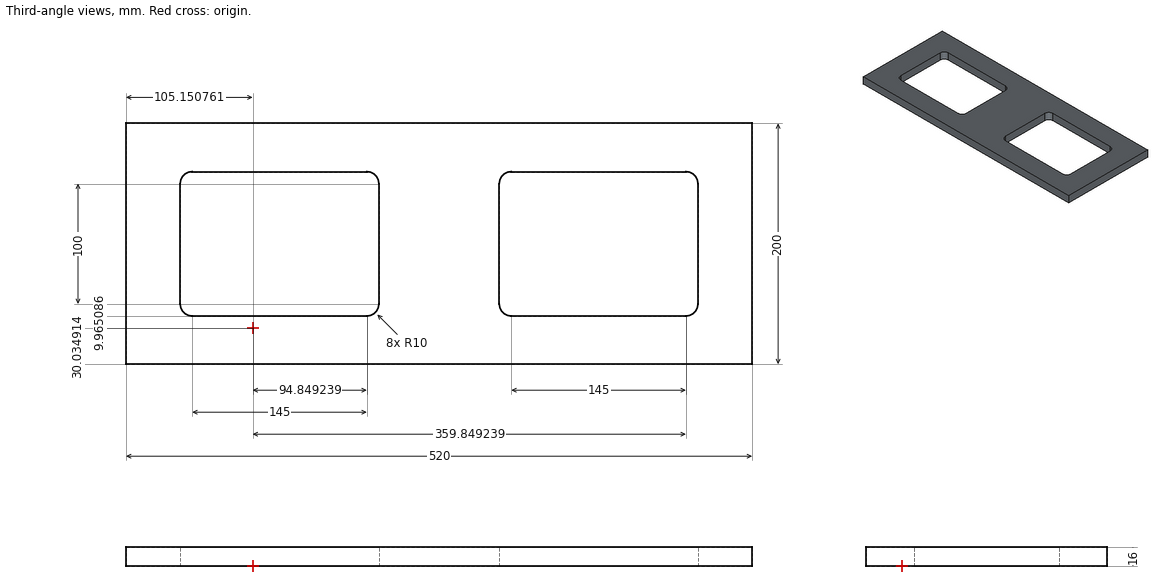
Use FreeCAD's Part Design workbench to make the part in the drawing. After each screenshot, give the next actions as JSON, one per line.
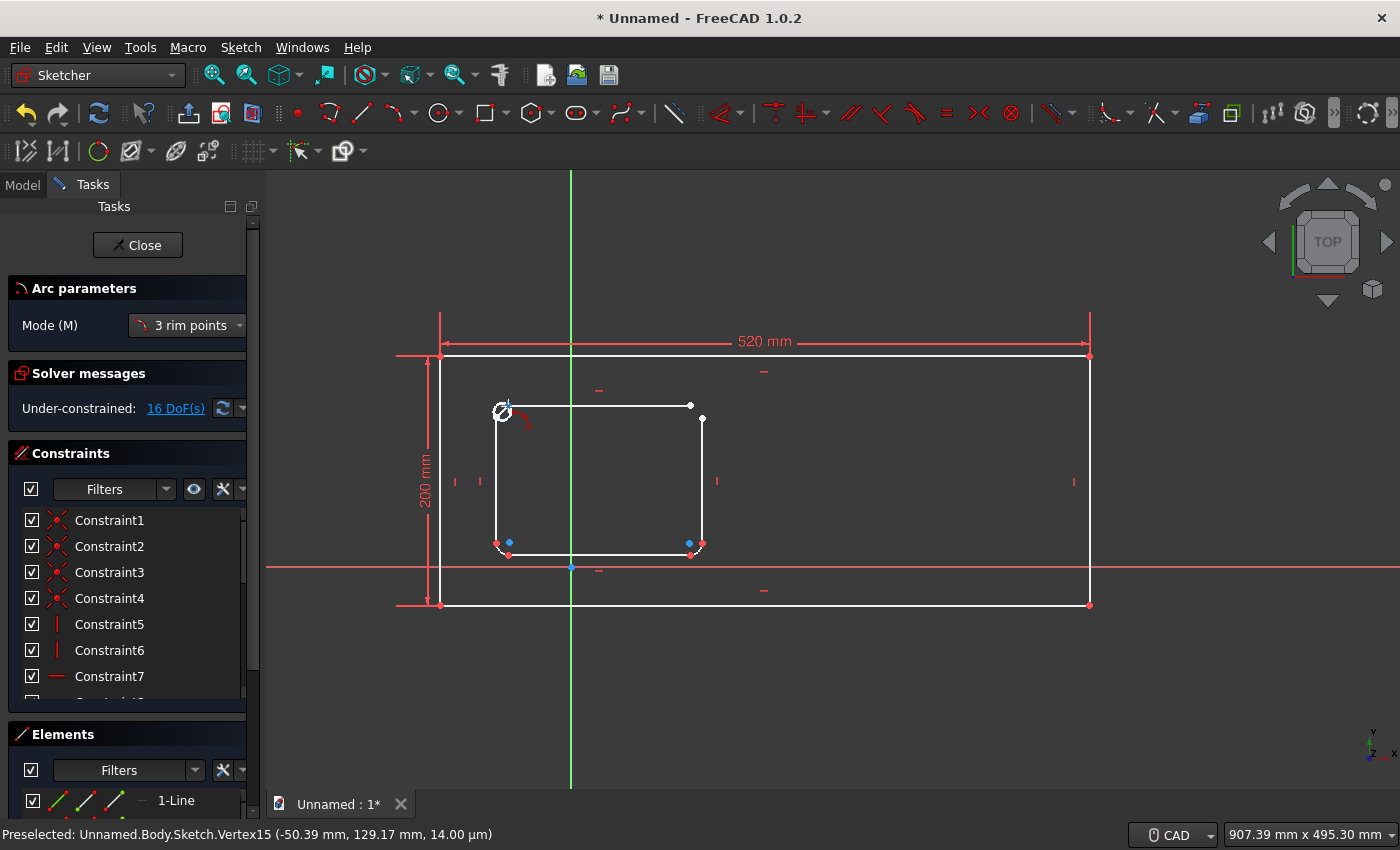
{"action": "scroll", "coordinate": [500, 408], "scroll_direction": "up", "scroll_amount": 8}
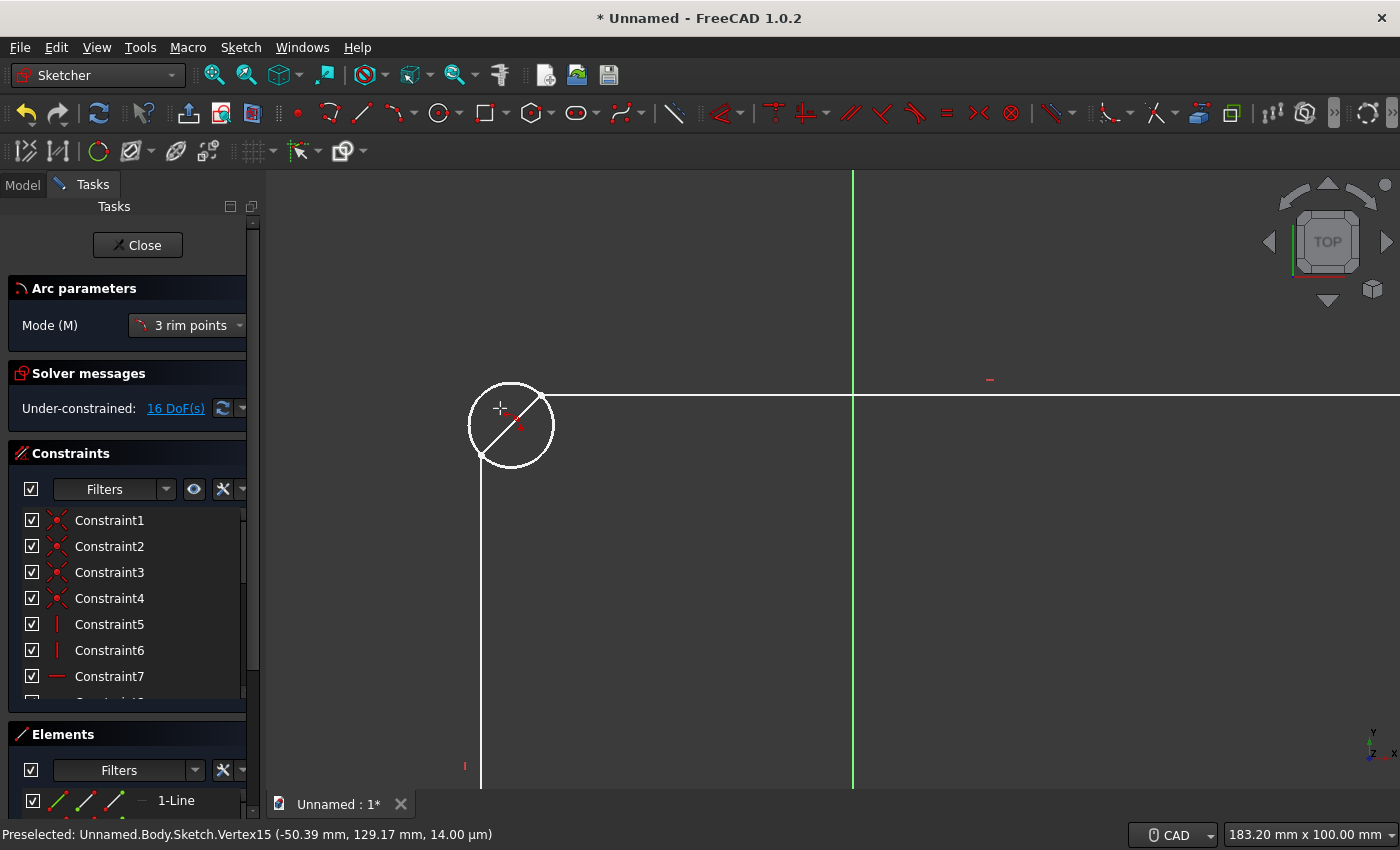
{"action": "left_click", "coordinate": [499, 409]}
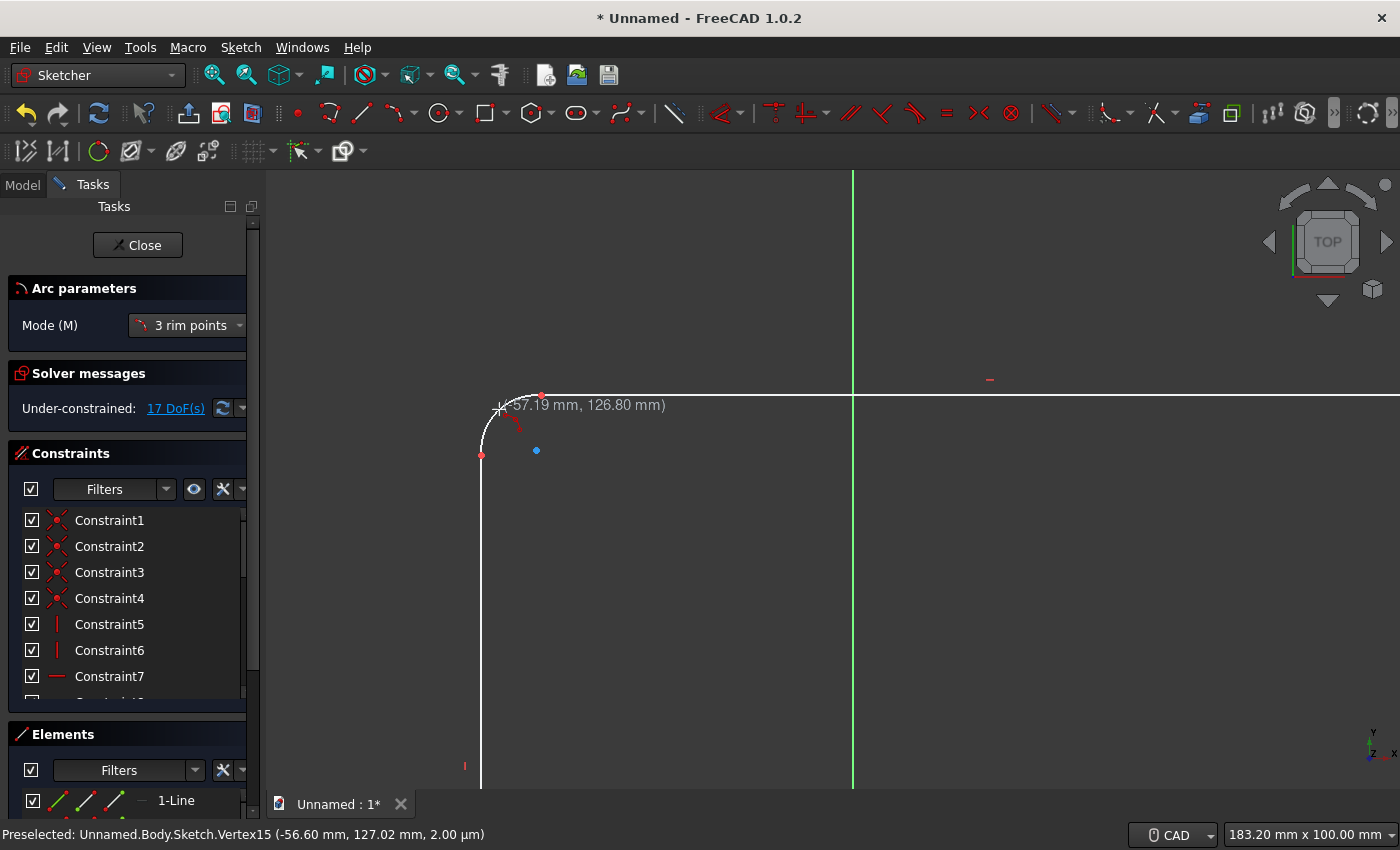
{"action": "scroll", "coordinate": [500, 408], "scroll_direction": "down", "scroll_amount": 8}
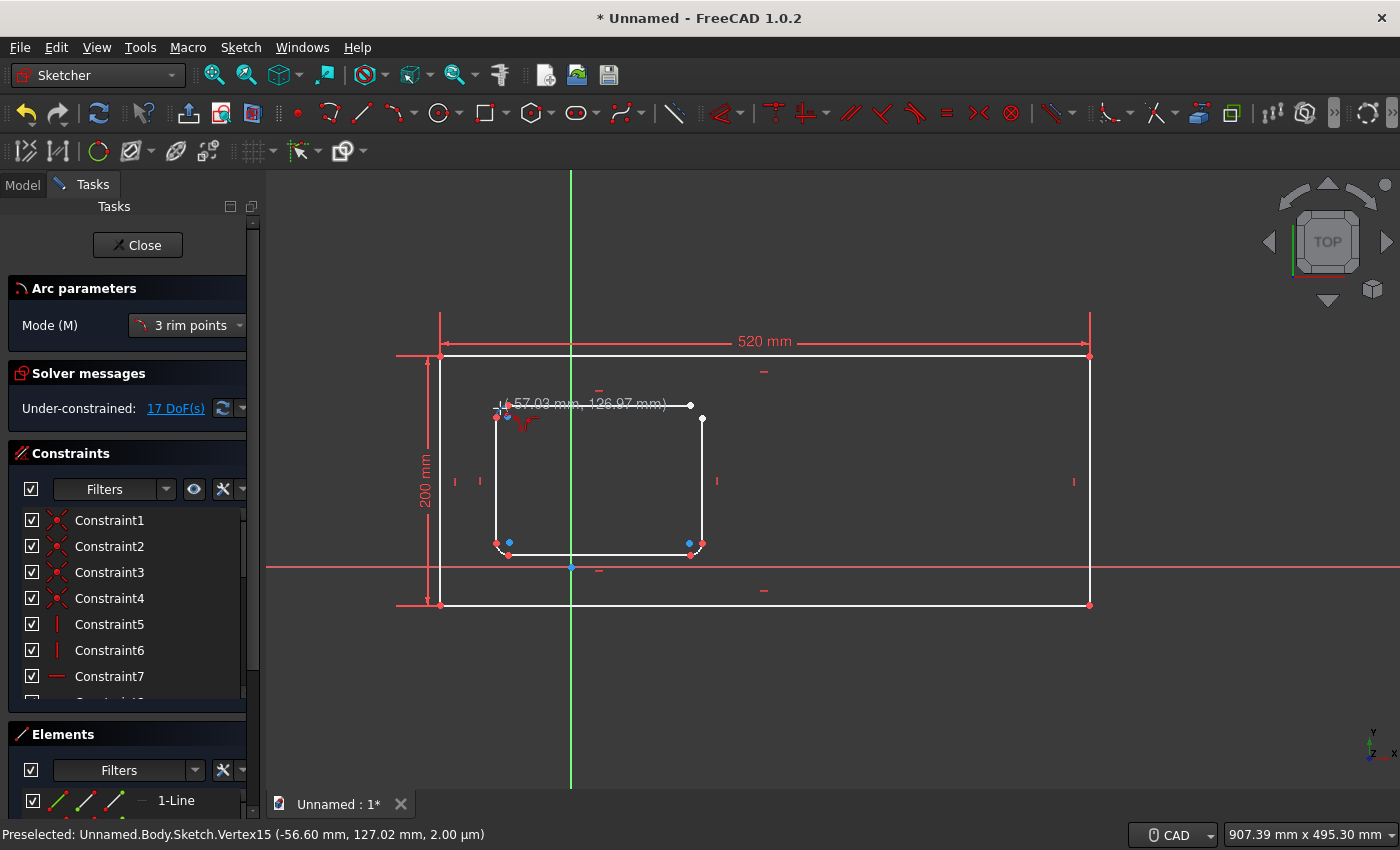
{"action": "left_click", "coordinate": [690, 406]}
{"action": "left_click", "coordinate": [702, 418]}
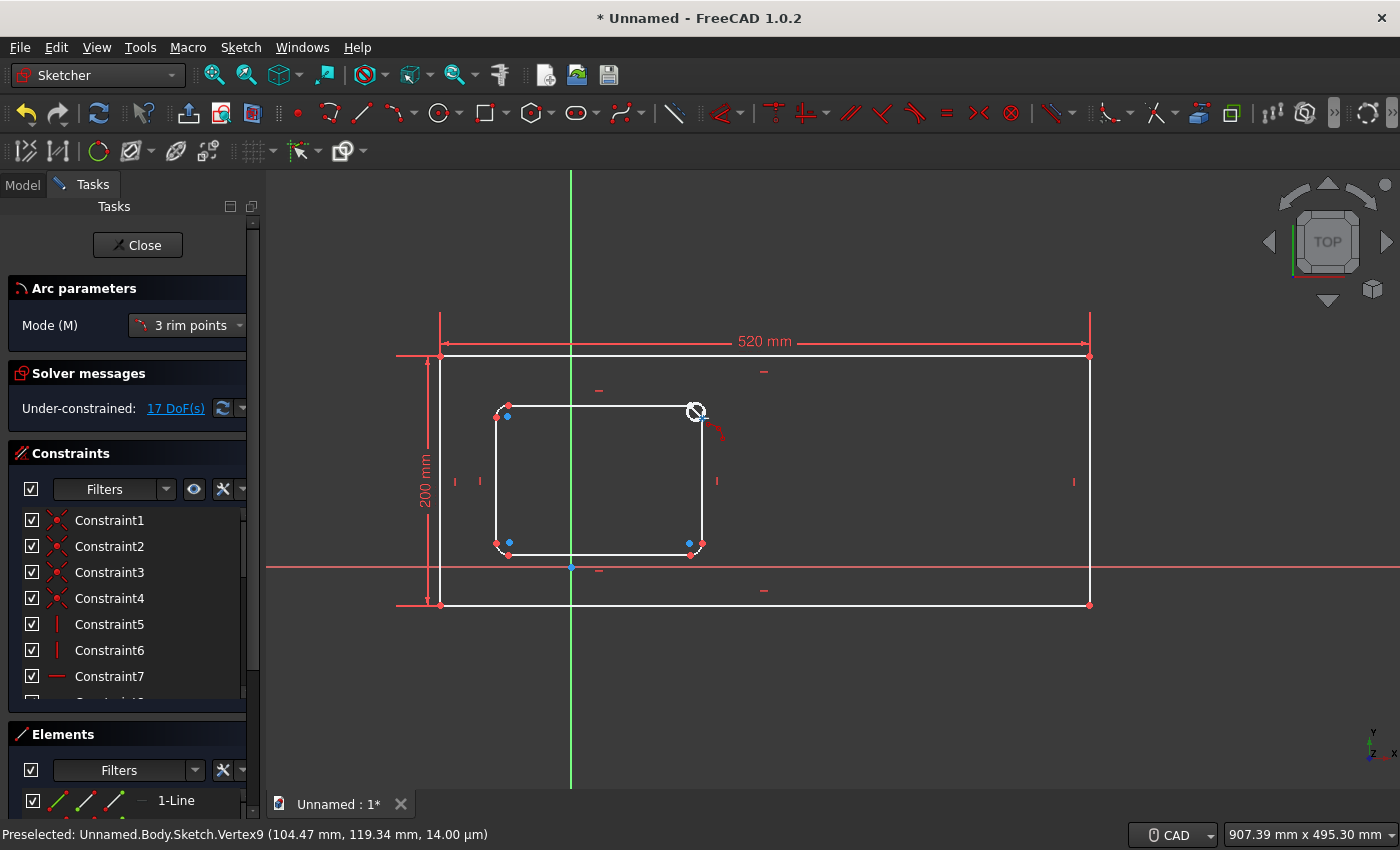
{"action": "scroll", "coordinate": [699, 408], "scroll_direction": "up", "scroll_amount": 8}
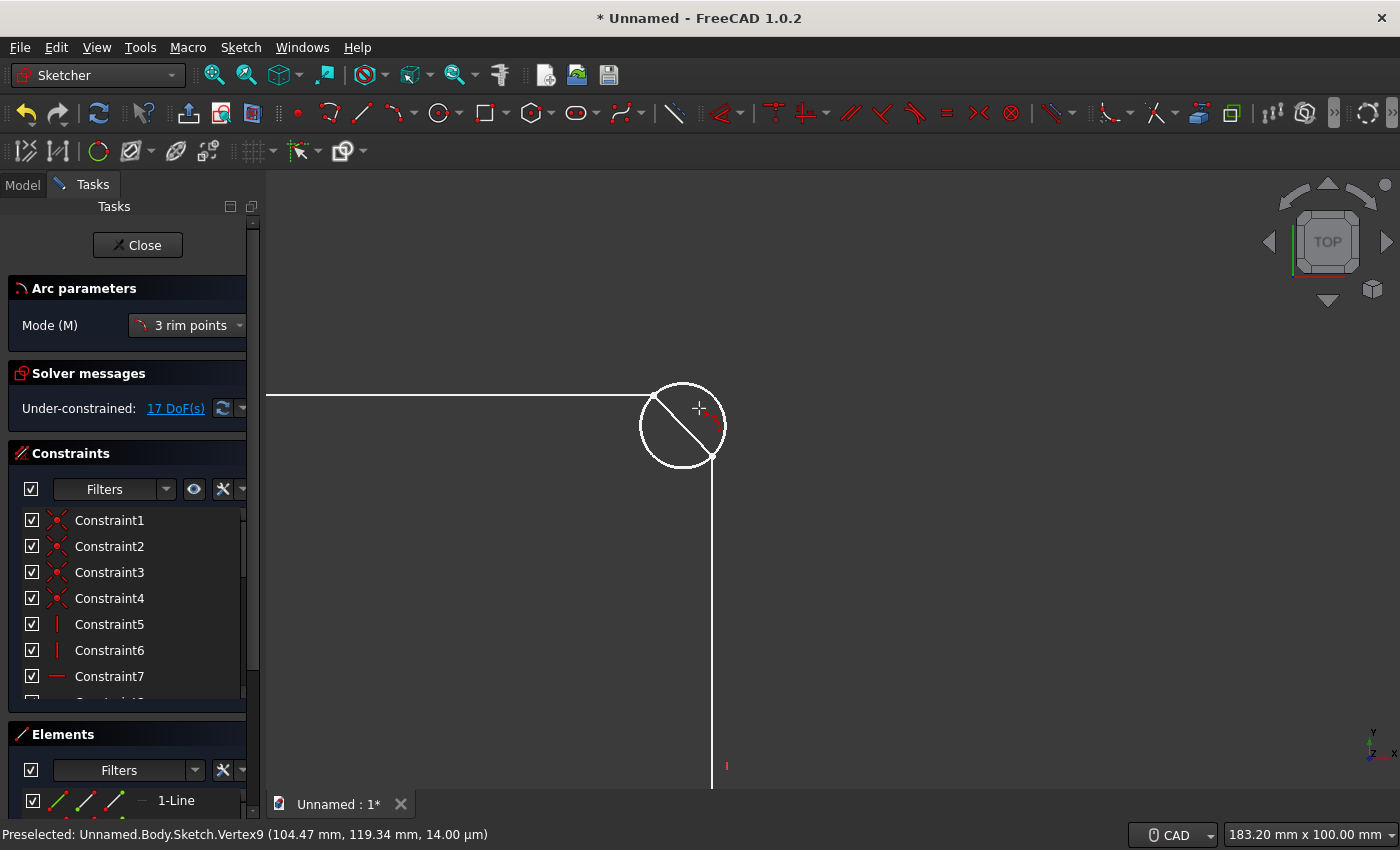
{"action": "left_click", "coordinate": [697, 409]}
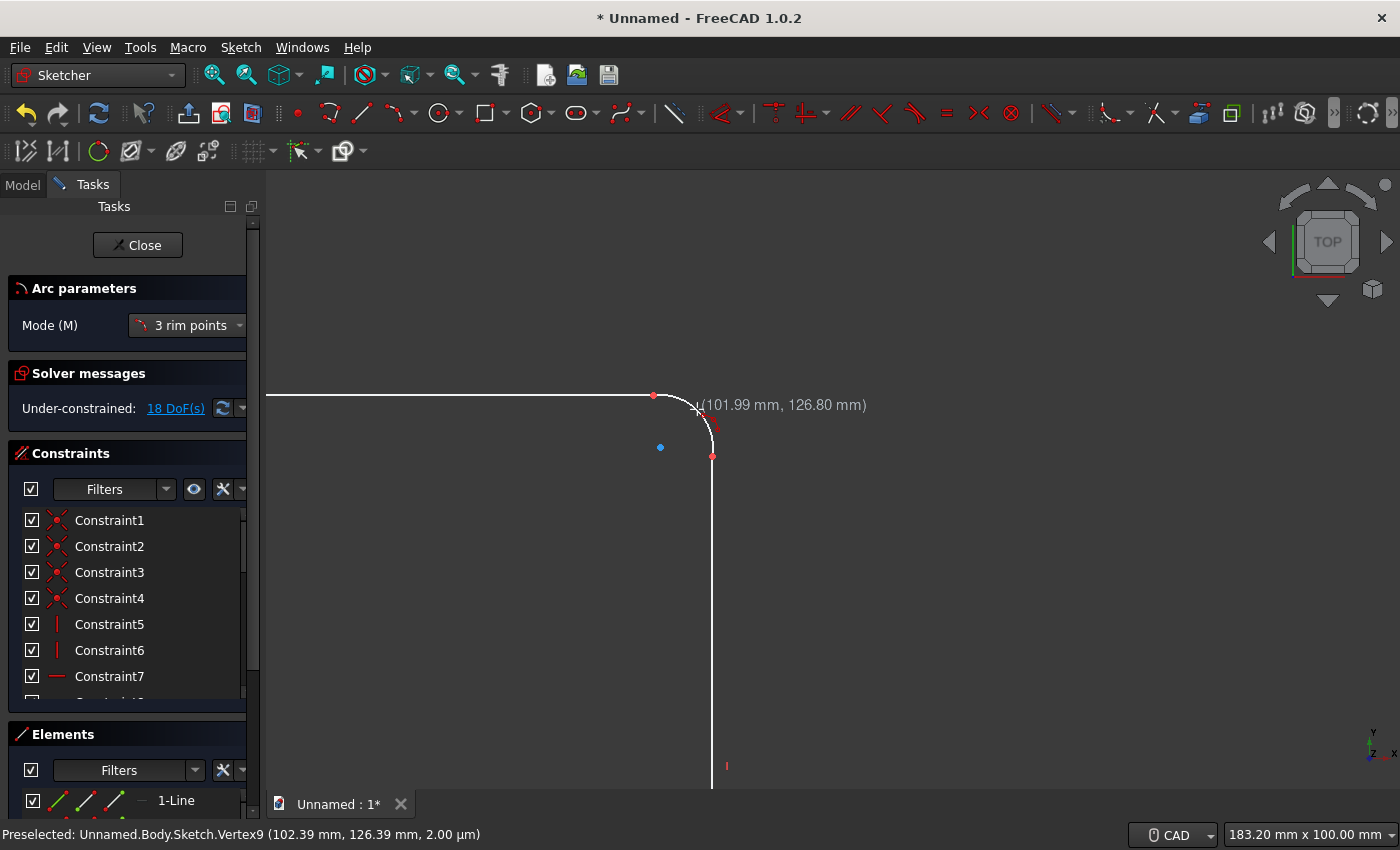
{"action": "key", "text": "g l"}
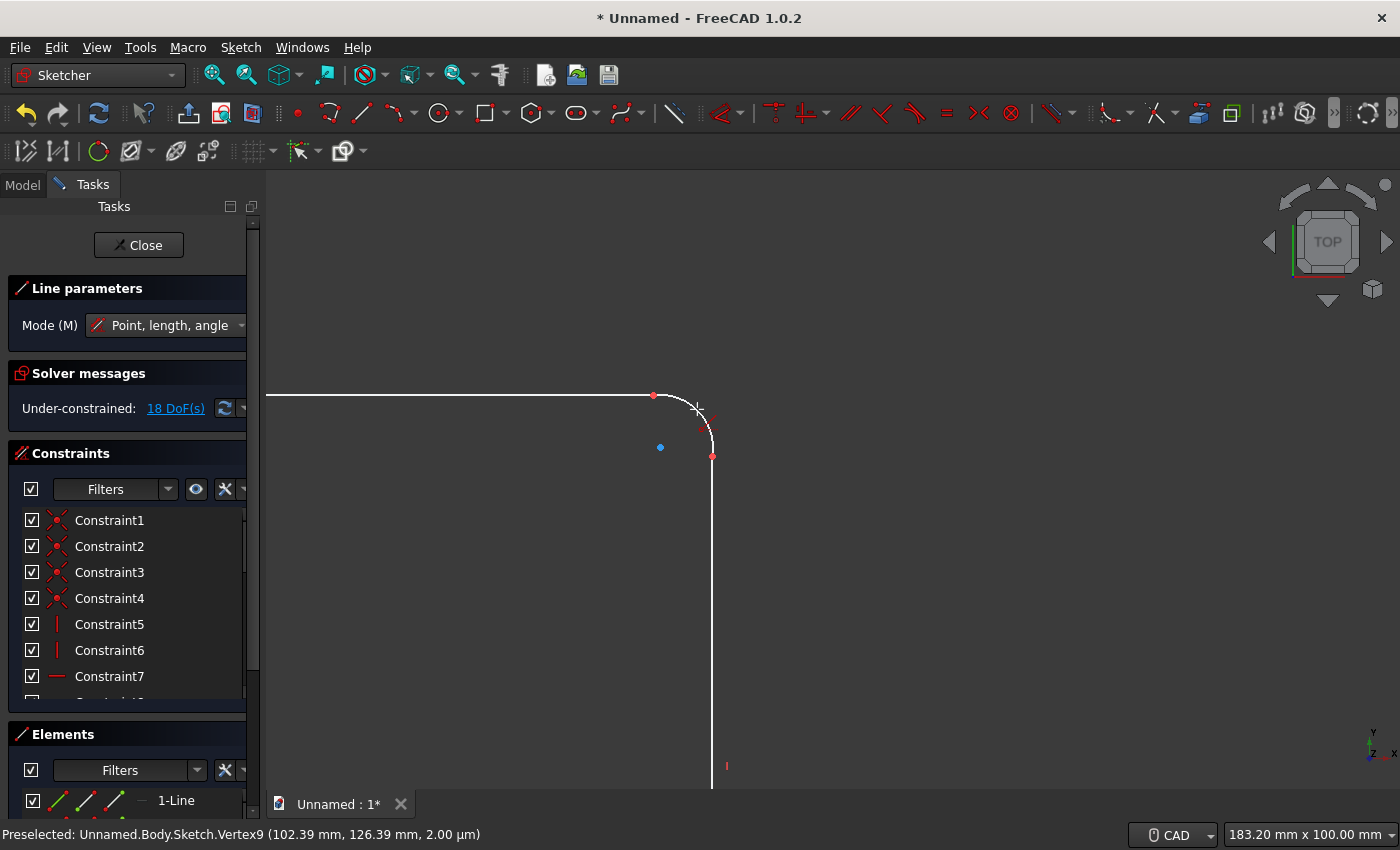
{"action": "scroll", "coordinate": [699, 408], "scroll_direction": "down", "scroll_amount": 8}